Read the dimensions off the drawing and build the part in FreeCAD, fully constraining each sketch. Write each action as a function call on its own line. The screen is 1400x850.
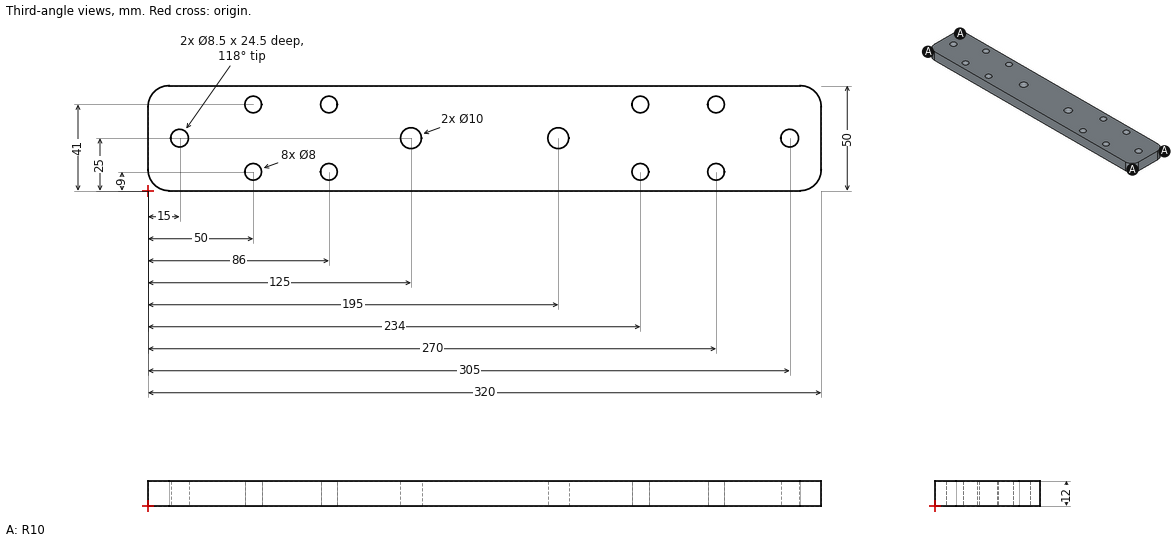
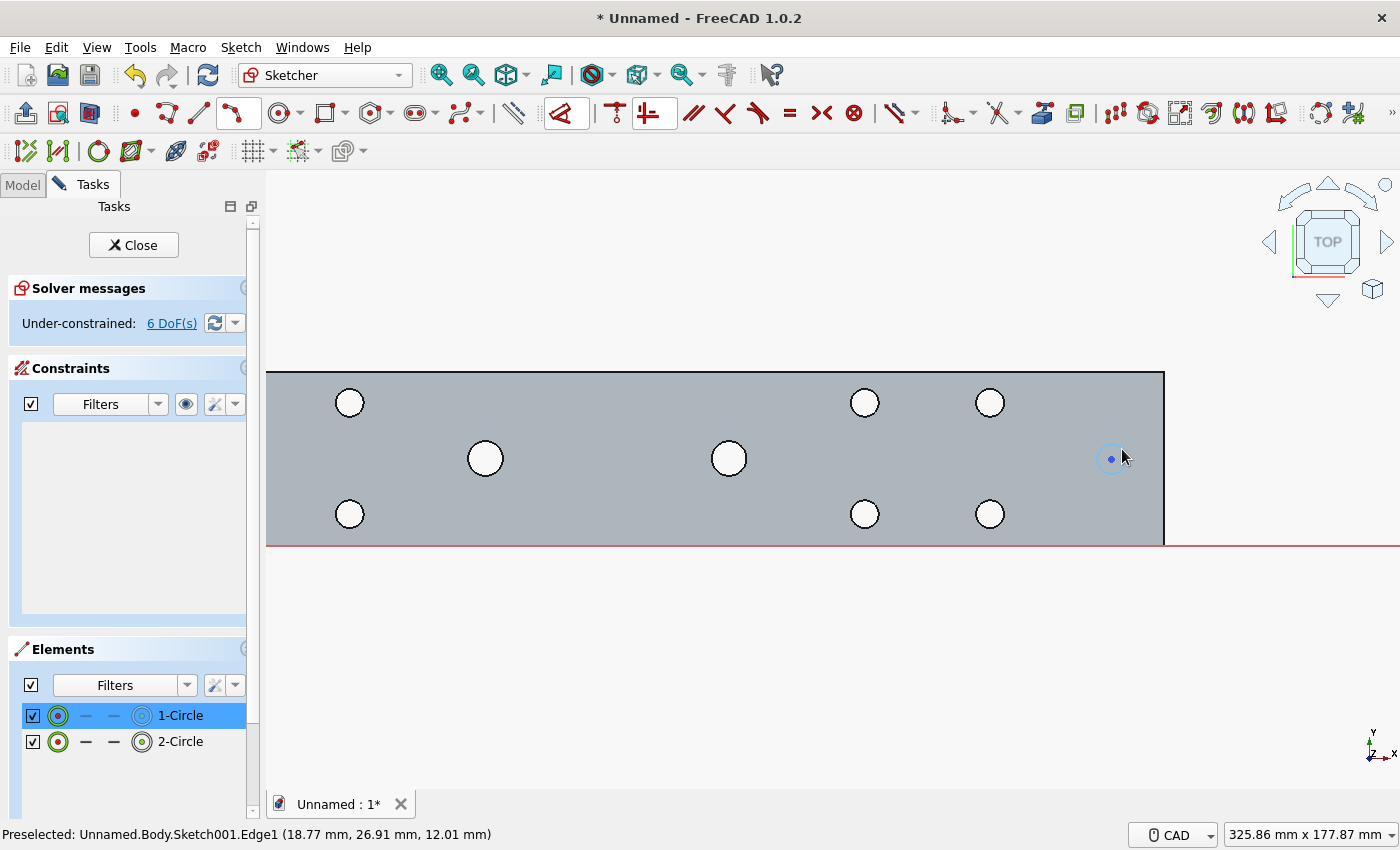
click(1122, 449)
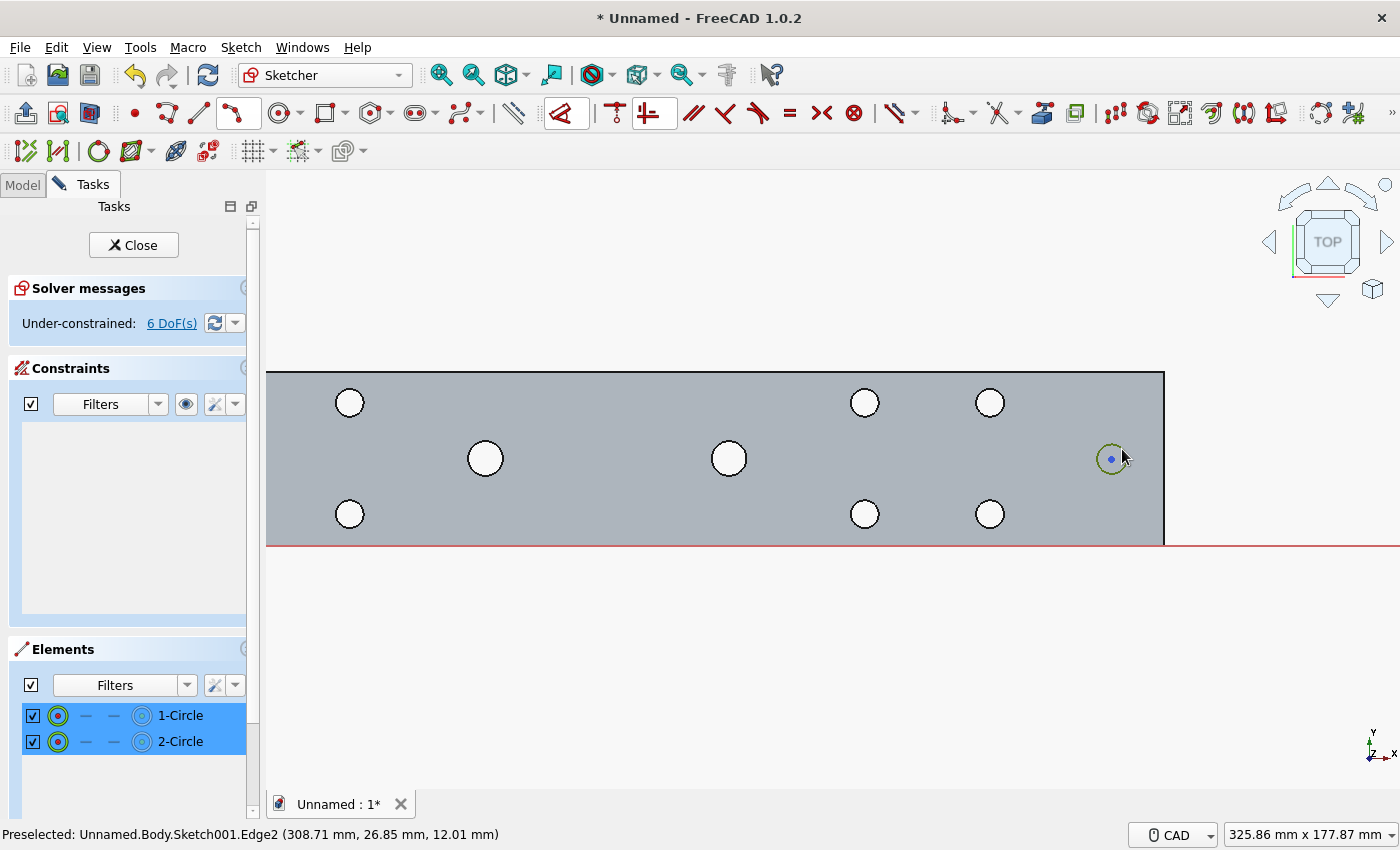
click(790, 114)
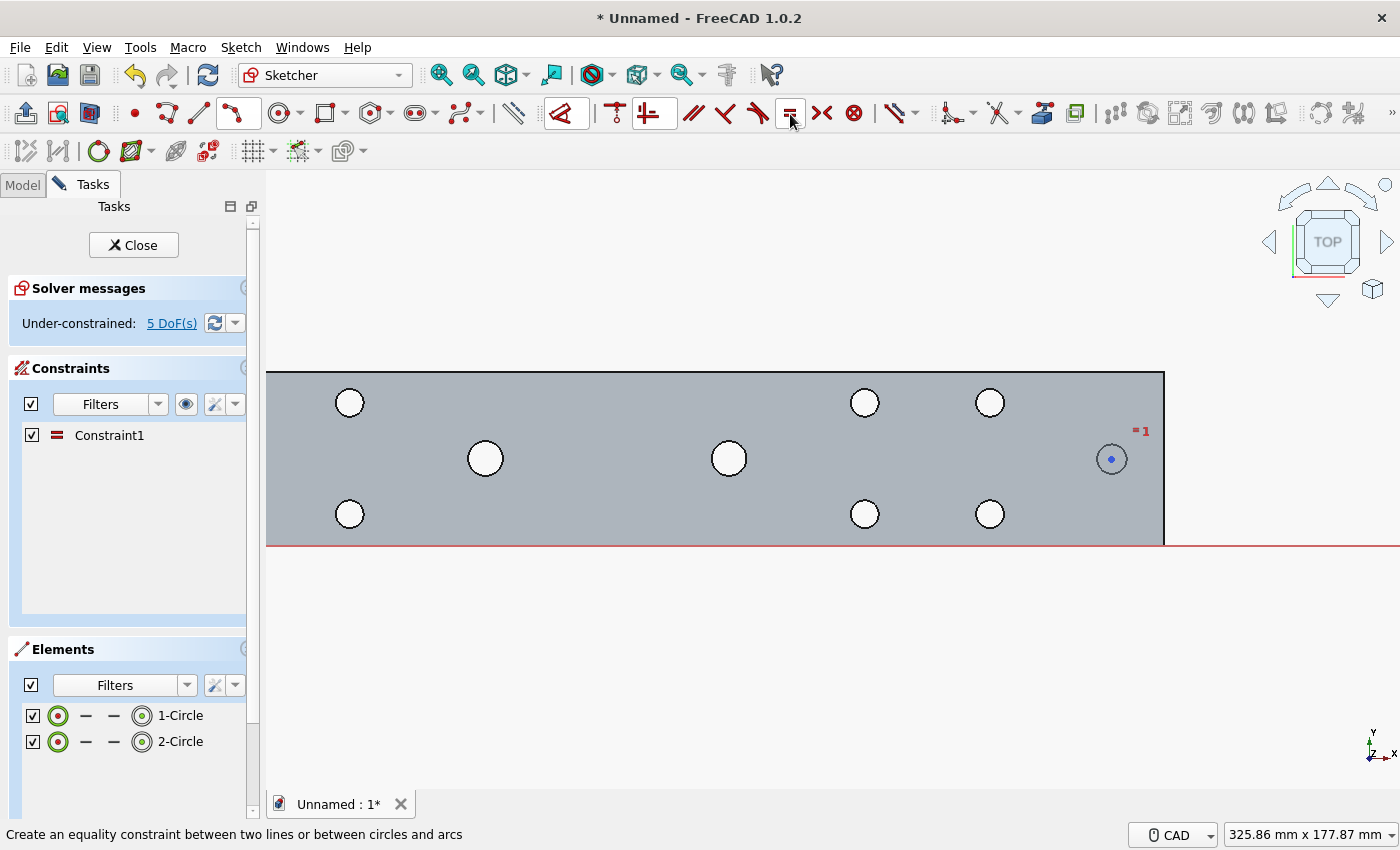
scroll(1122, 449, down, 2)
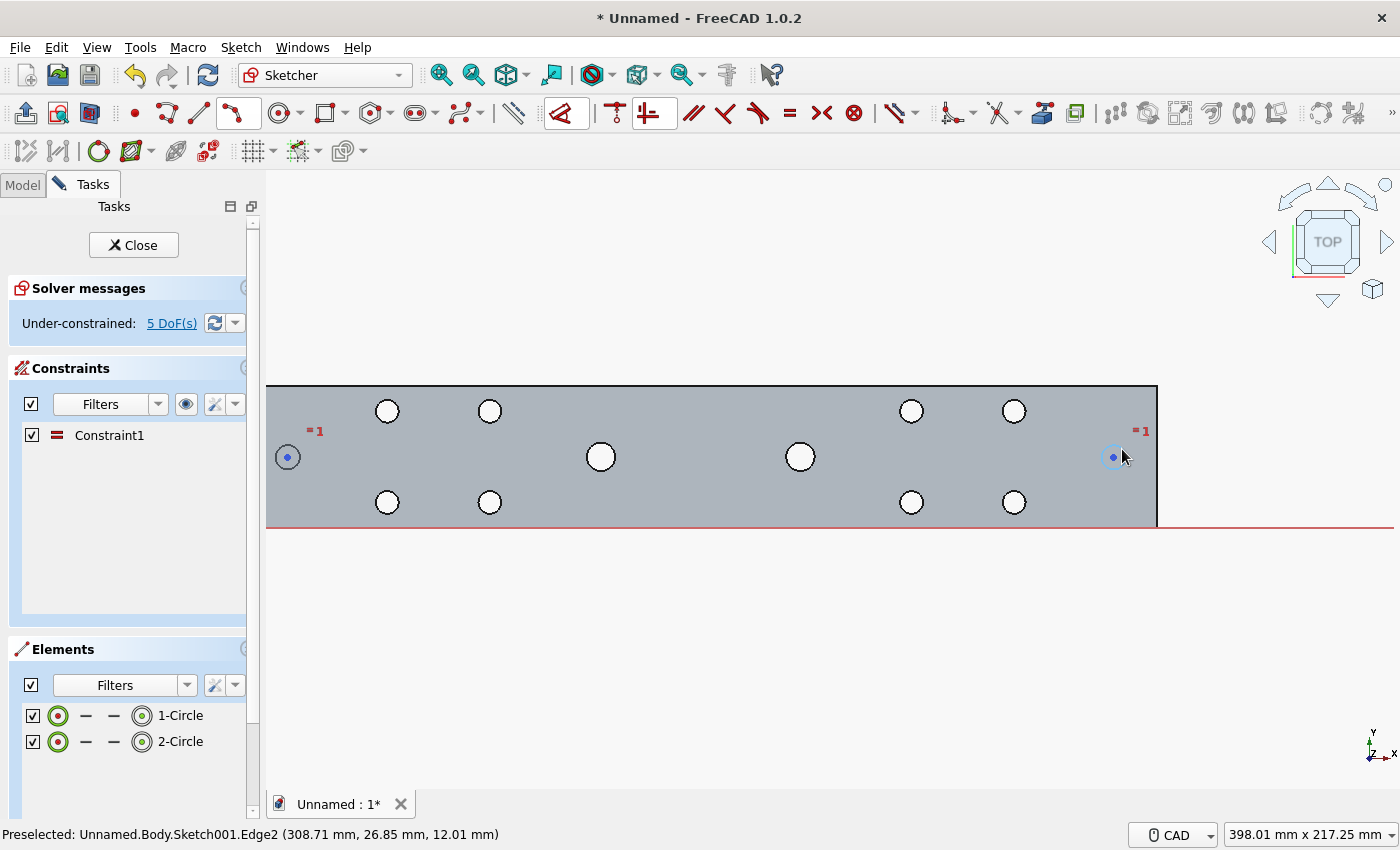
scroll(446, 449, up, 4)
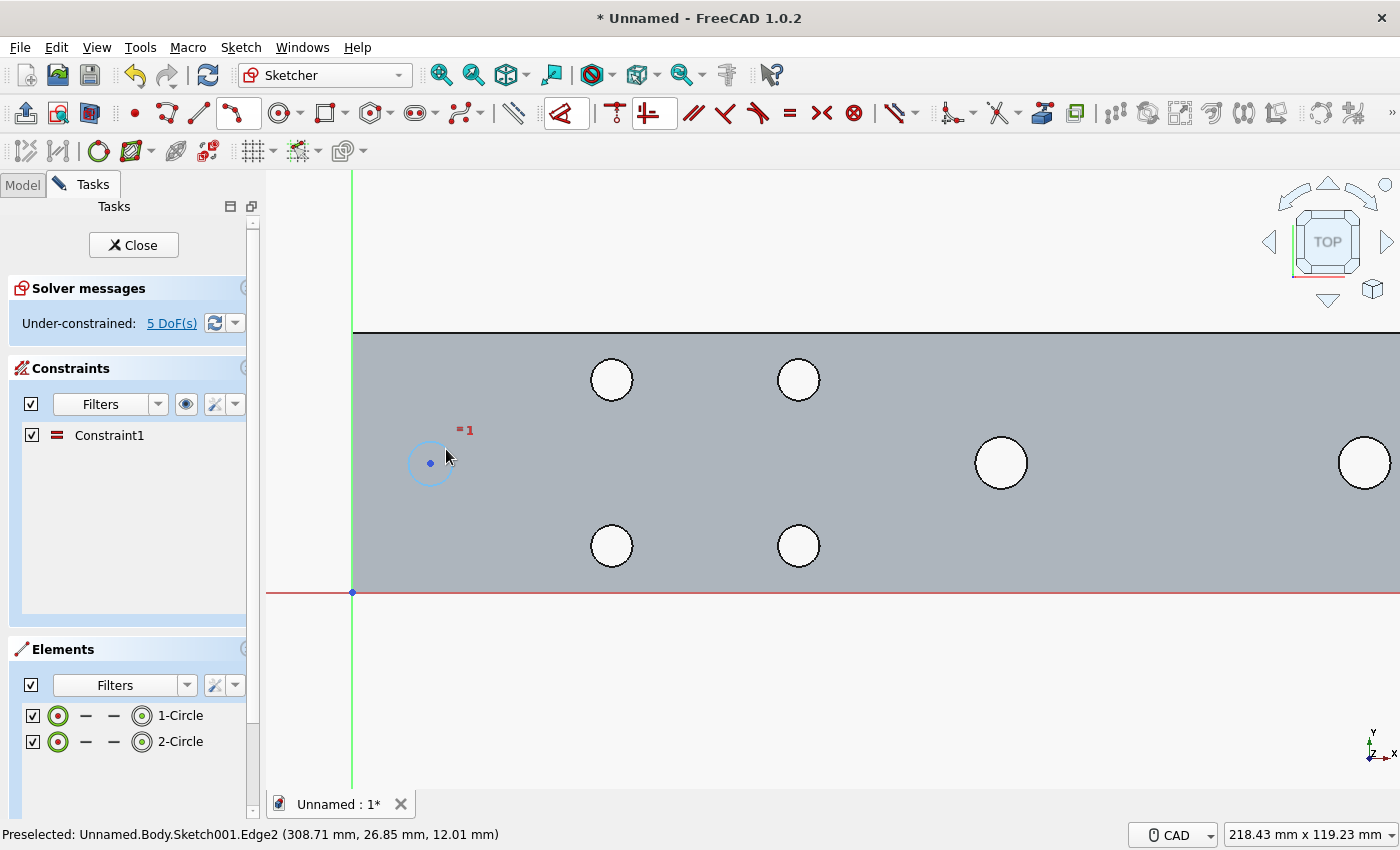
click(446, 448)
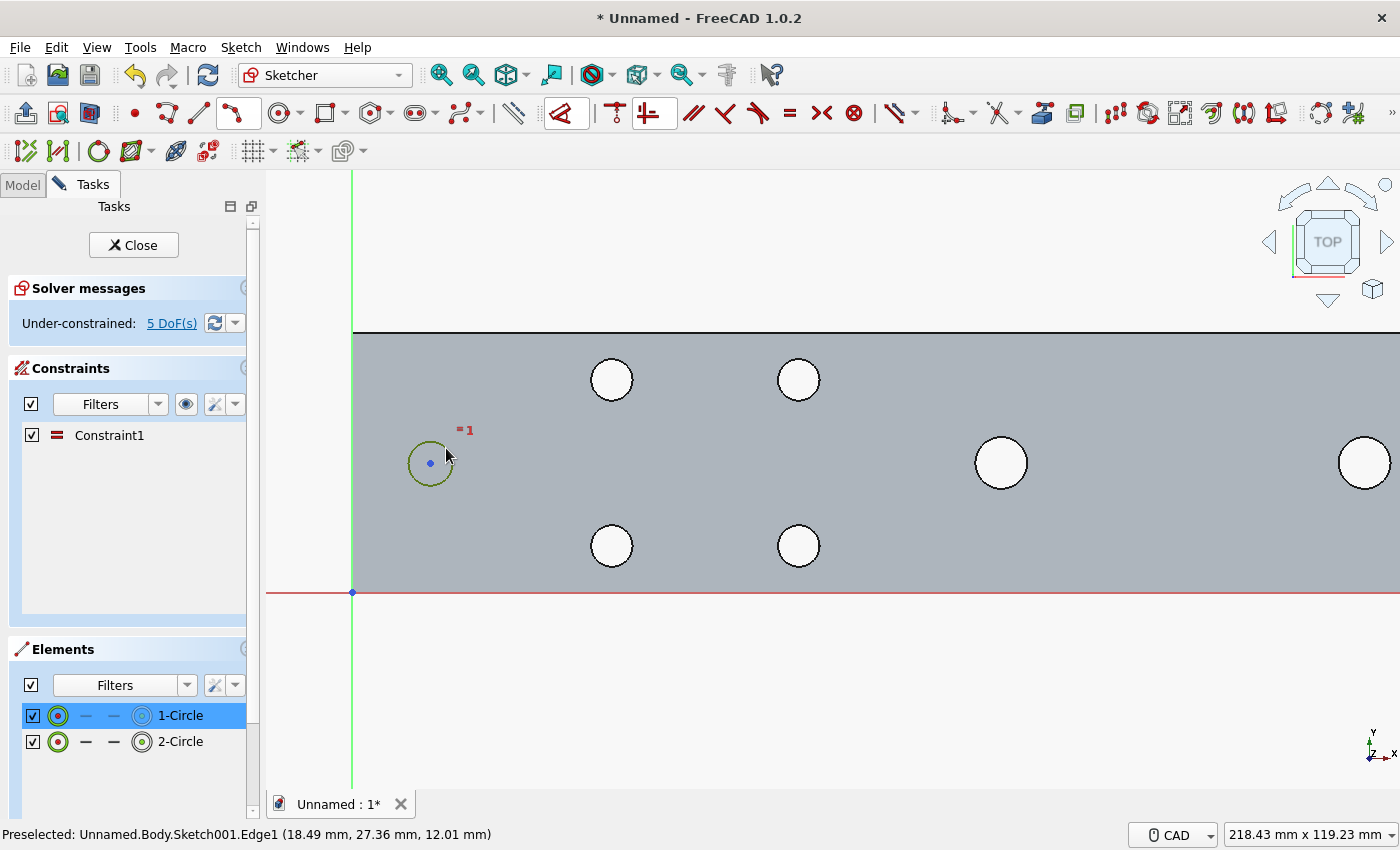
click(584, 114)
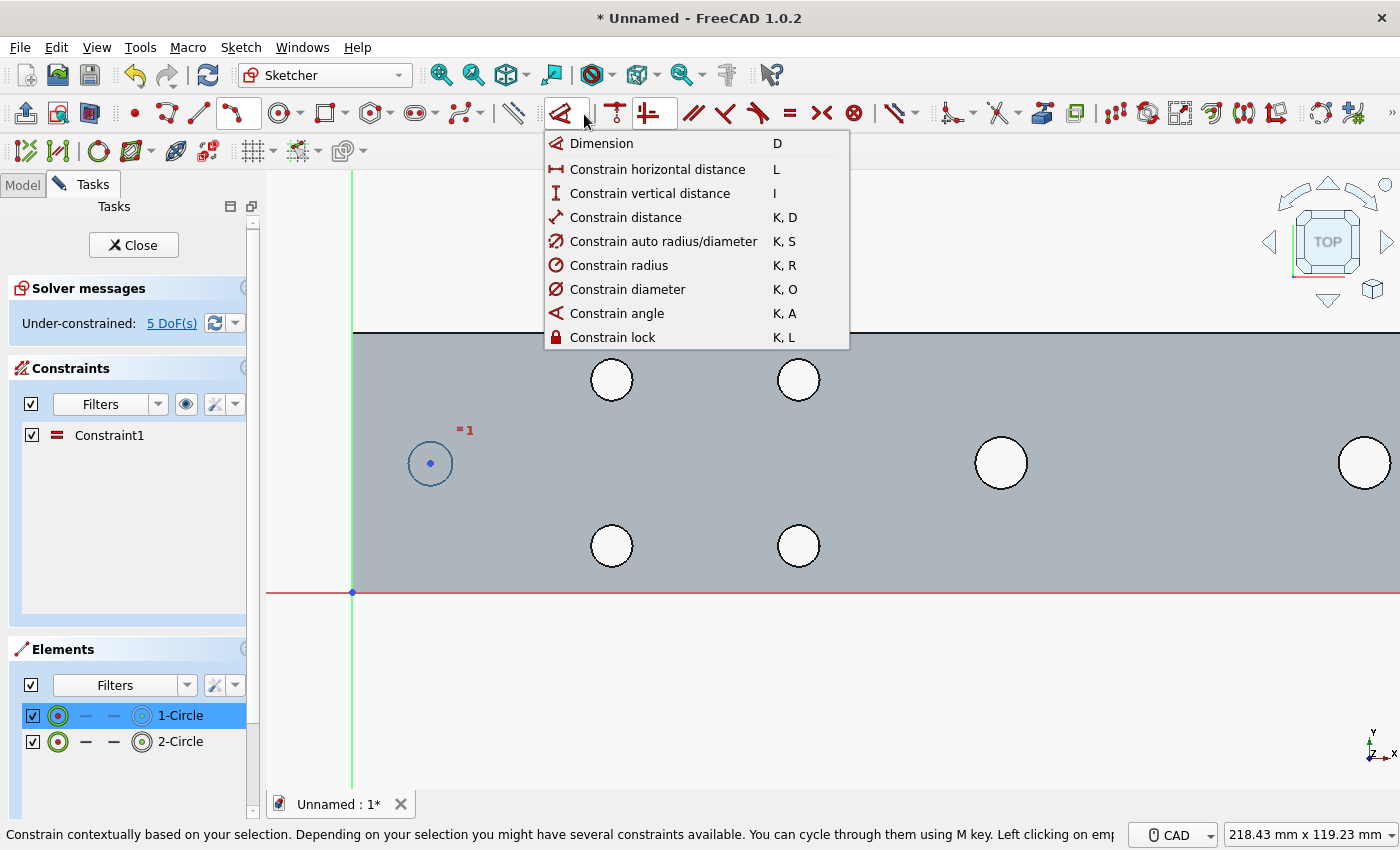
click(697, 289)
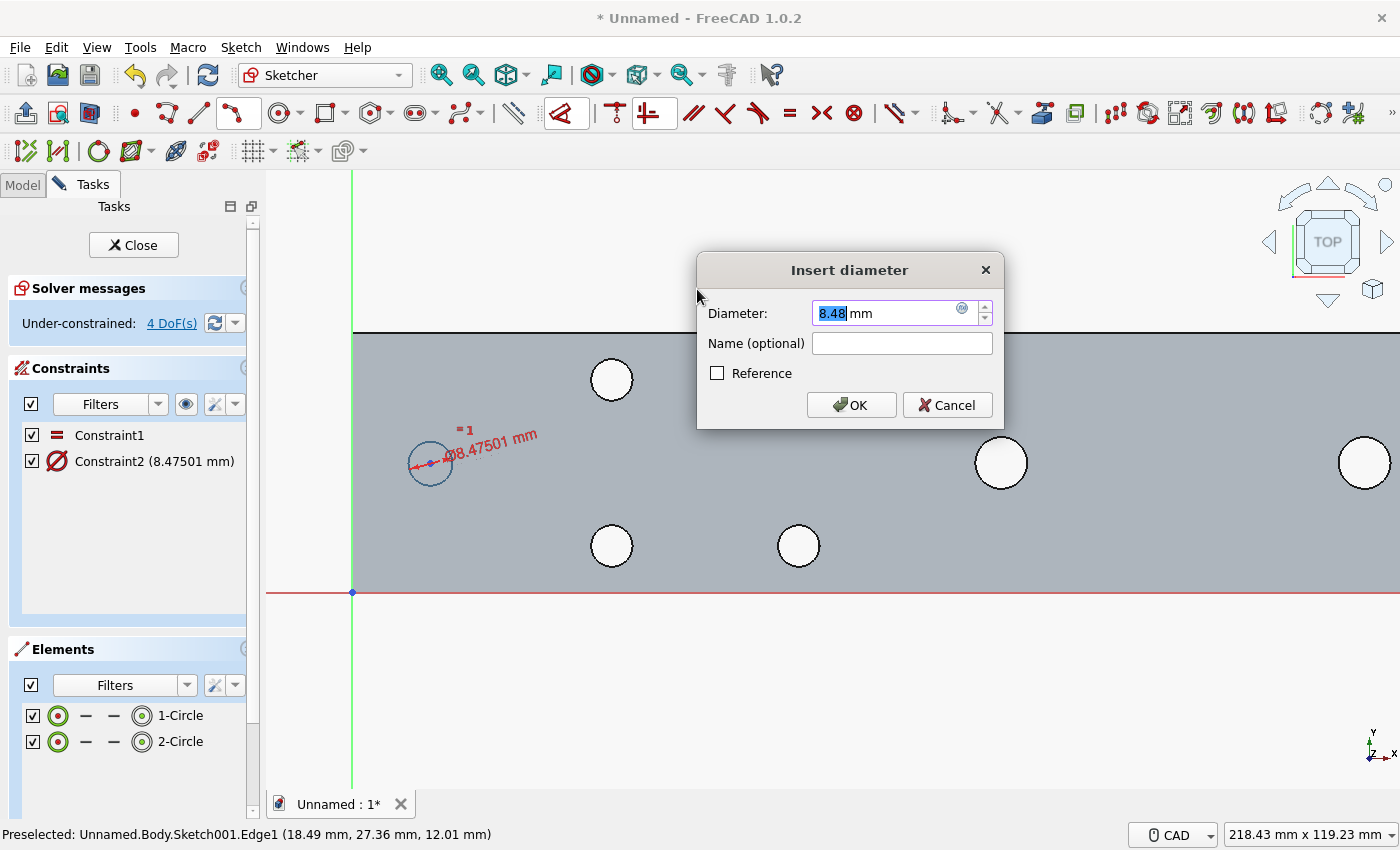
text(8.5)
key(Return)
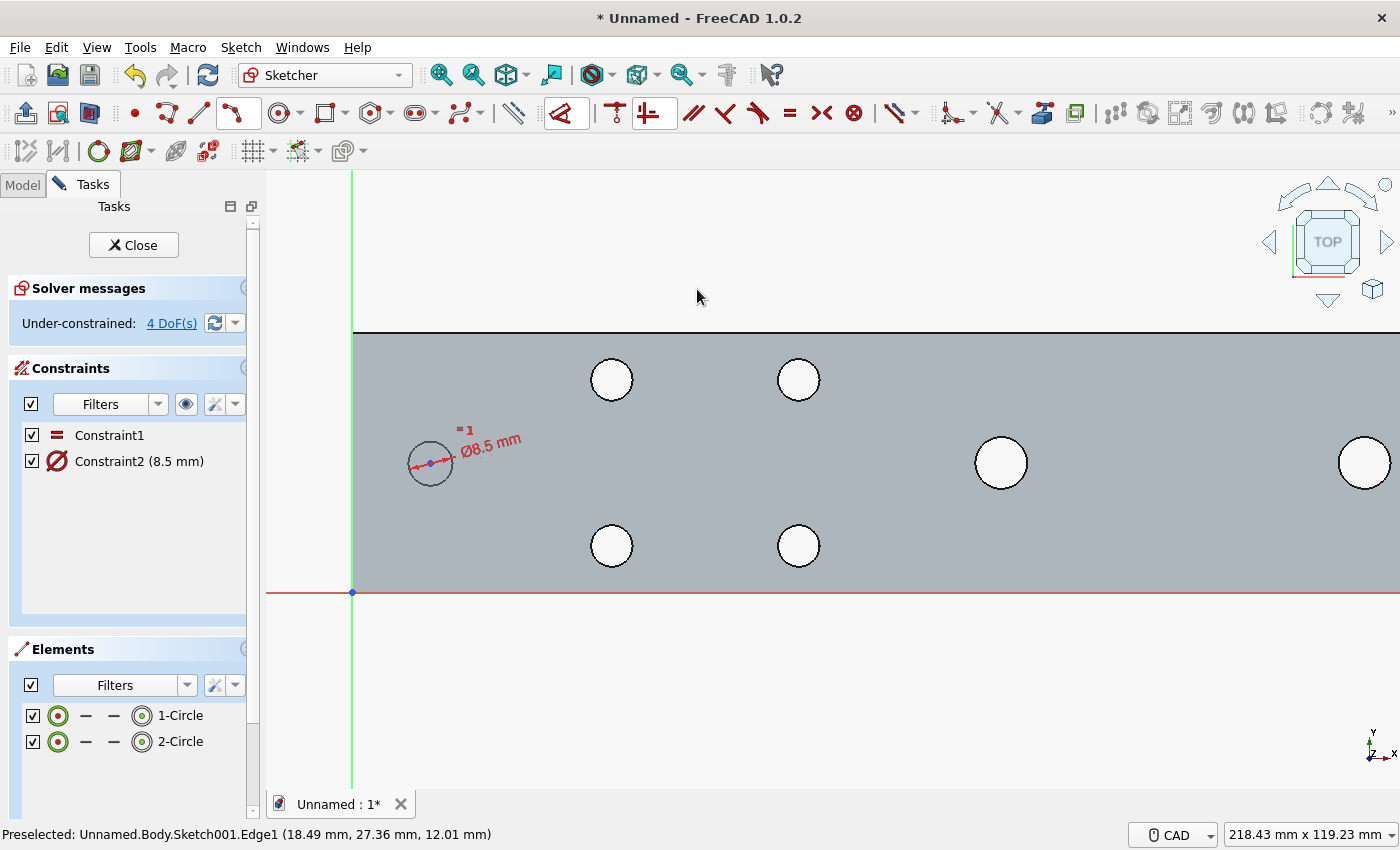
click(430, 464)